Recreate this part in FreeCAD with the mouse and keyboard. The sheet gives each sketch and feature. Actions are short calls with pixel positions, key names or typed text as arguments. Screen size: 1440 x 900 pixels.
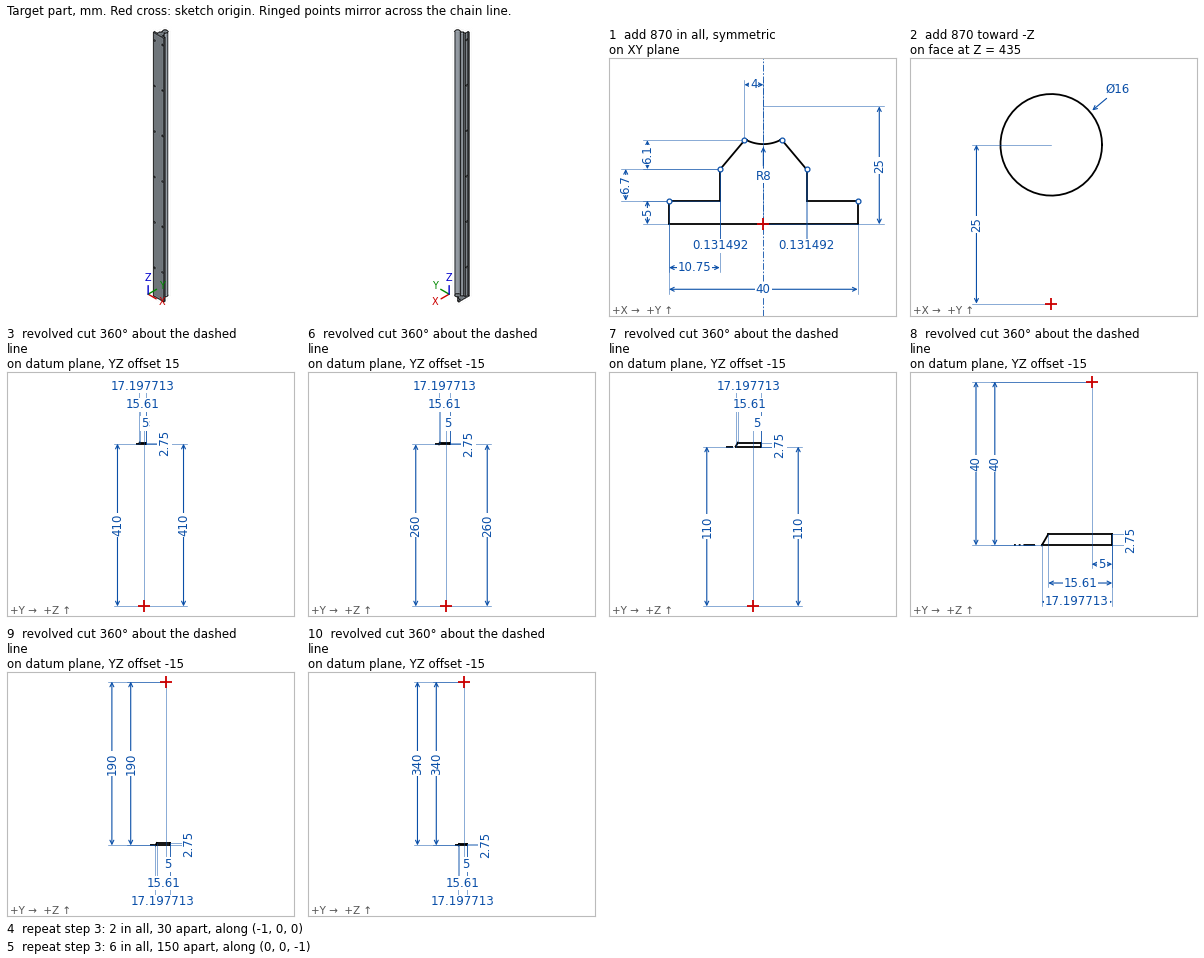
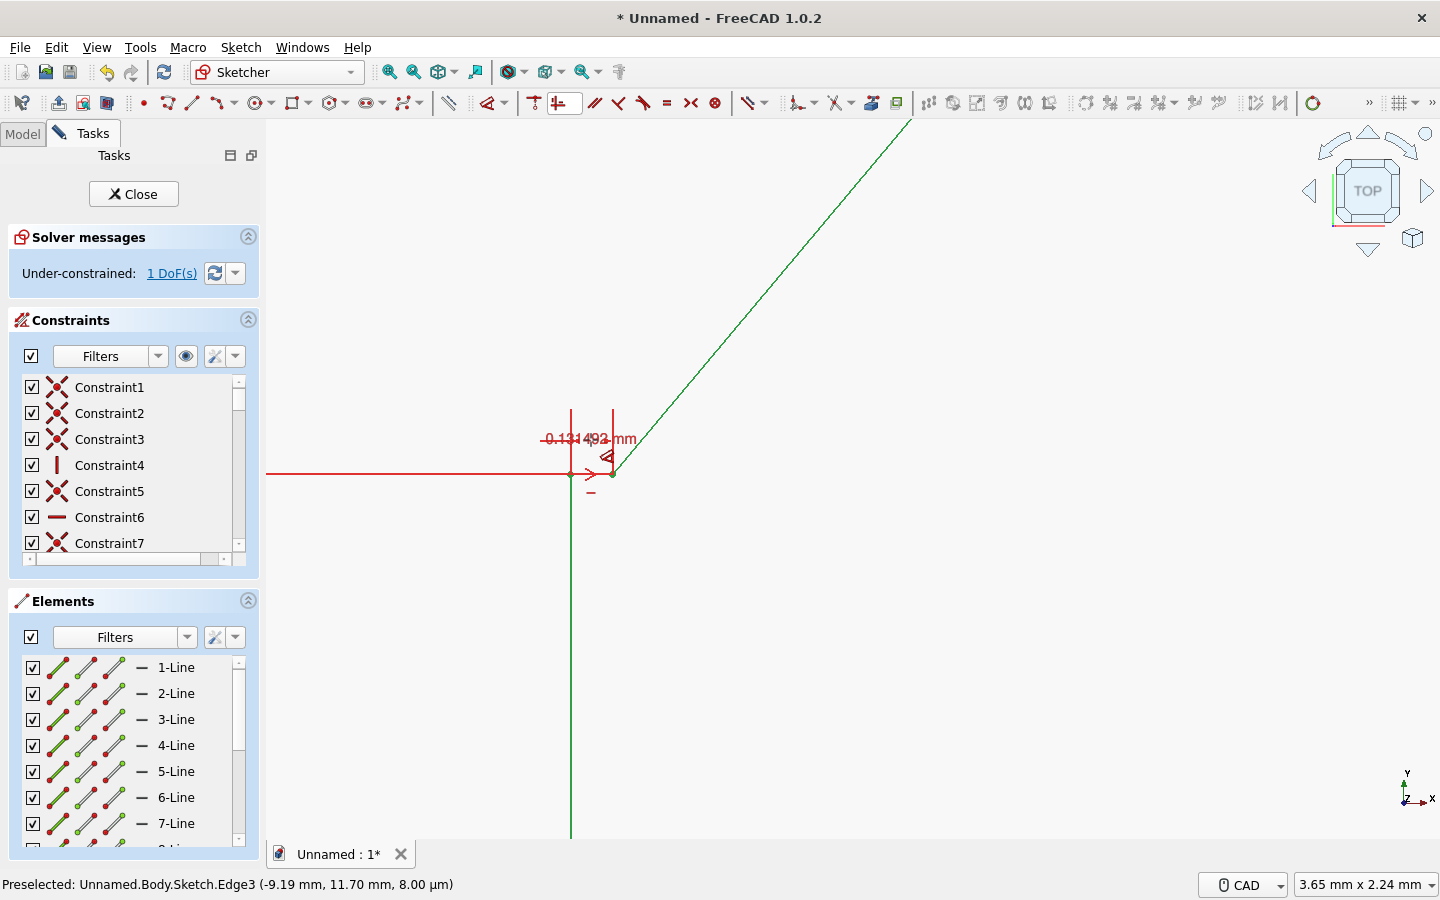
scroll(640, 432, down, 15)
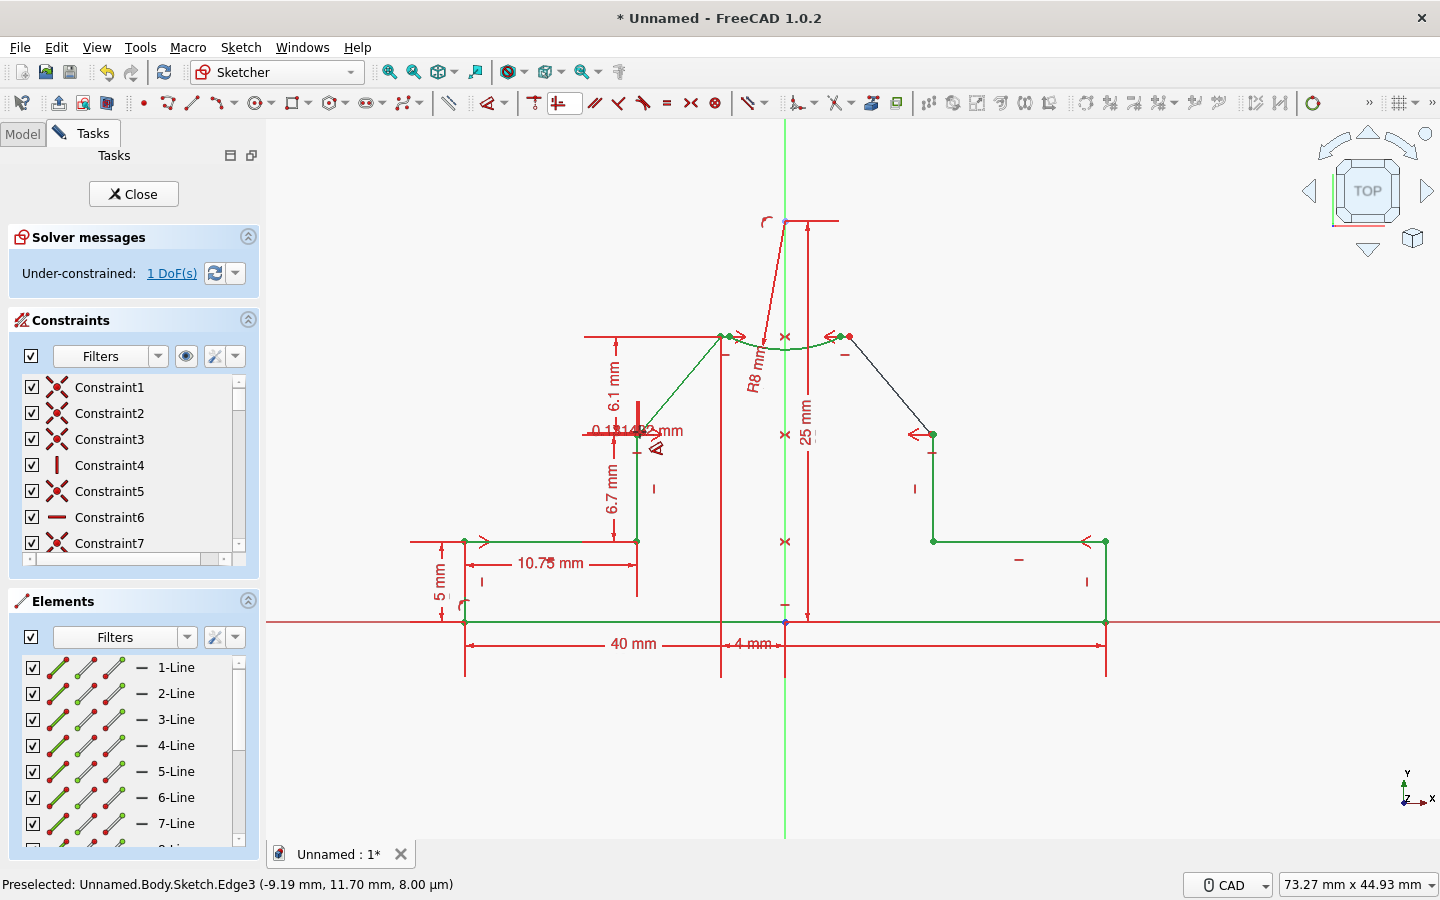
scroll(933, 435, up, 15)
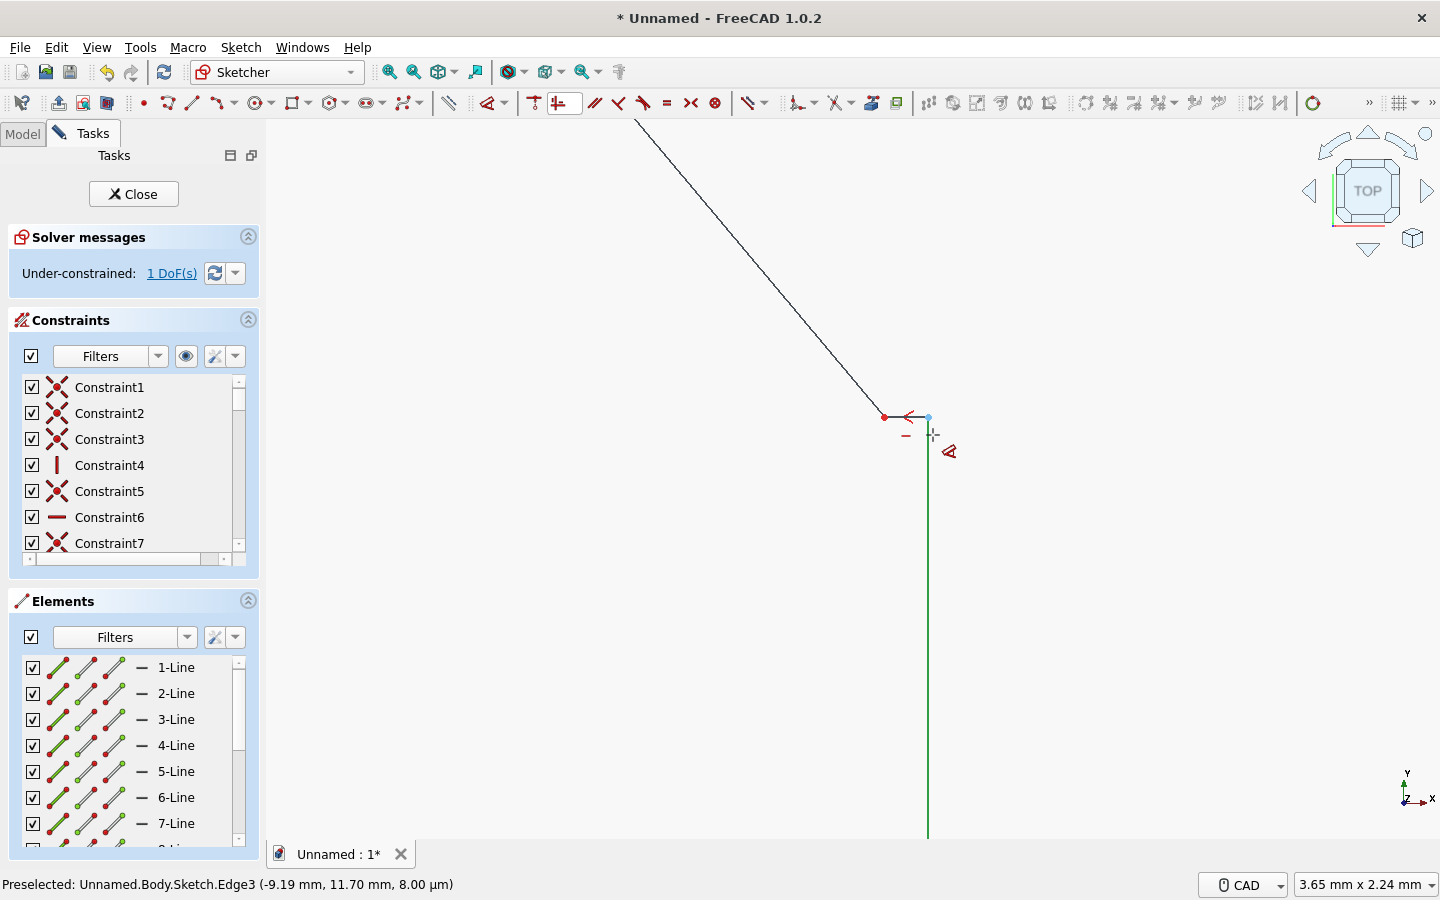
click(915, 417)
click(906, 383)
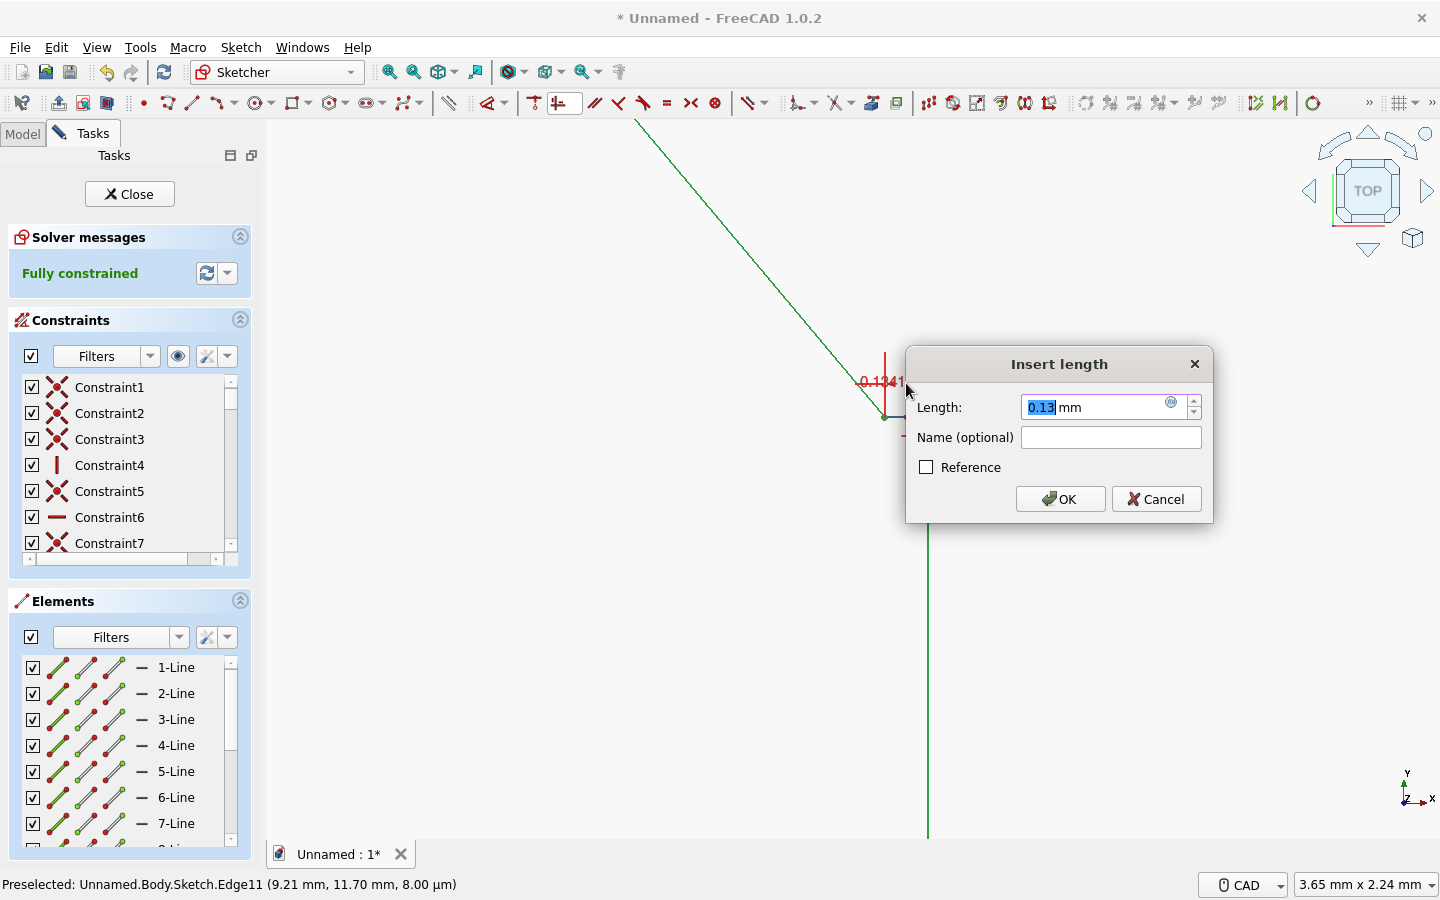
text(0.131492)
key(Return)
key(Escape)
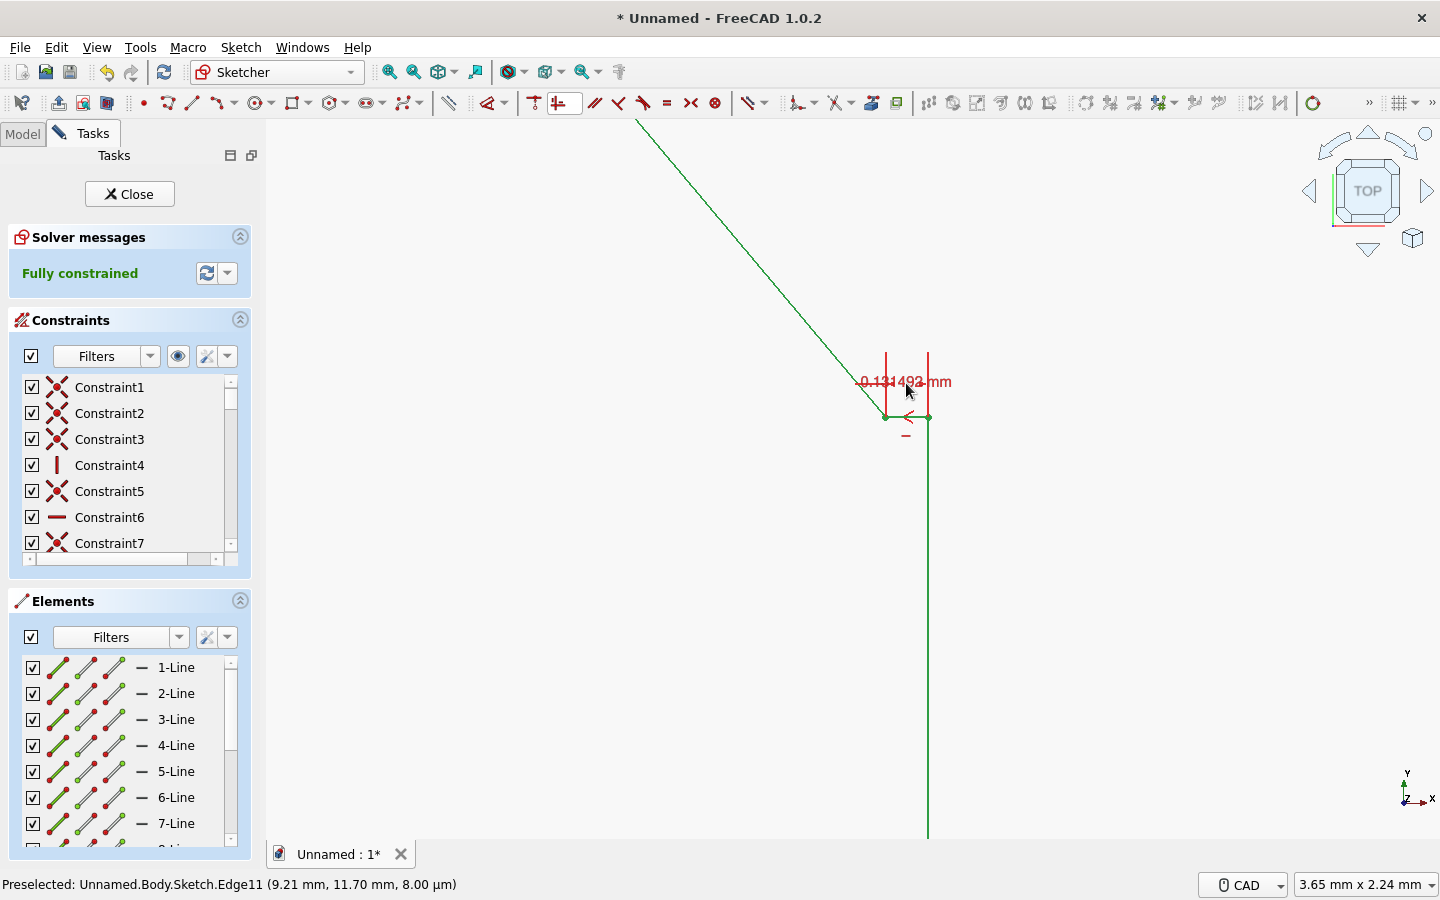
click(130, 194)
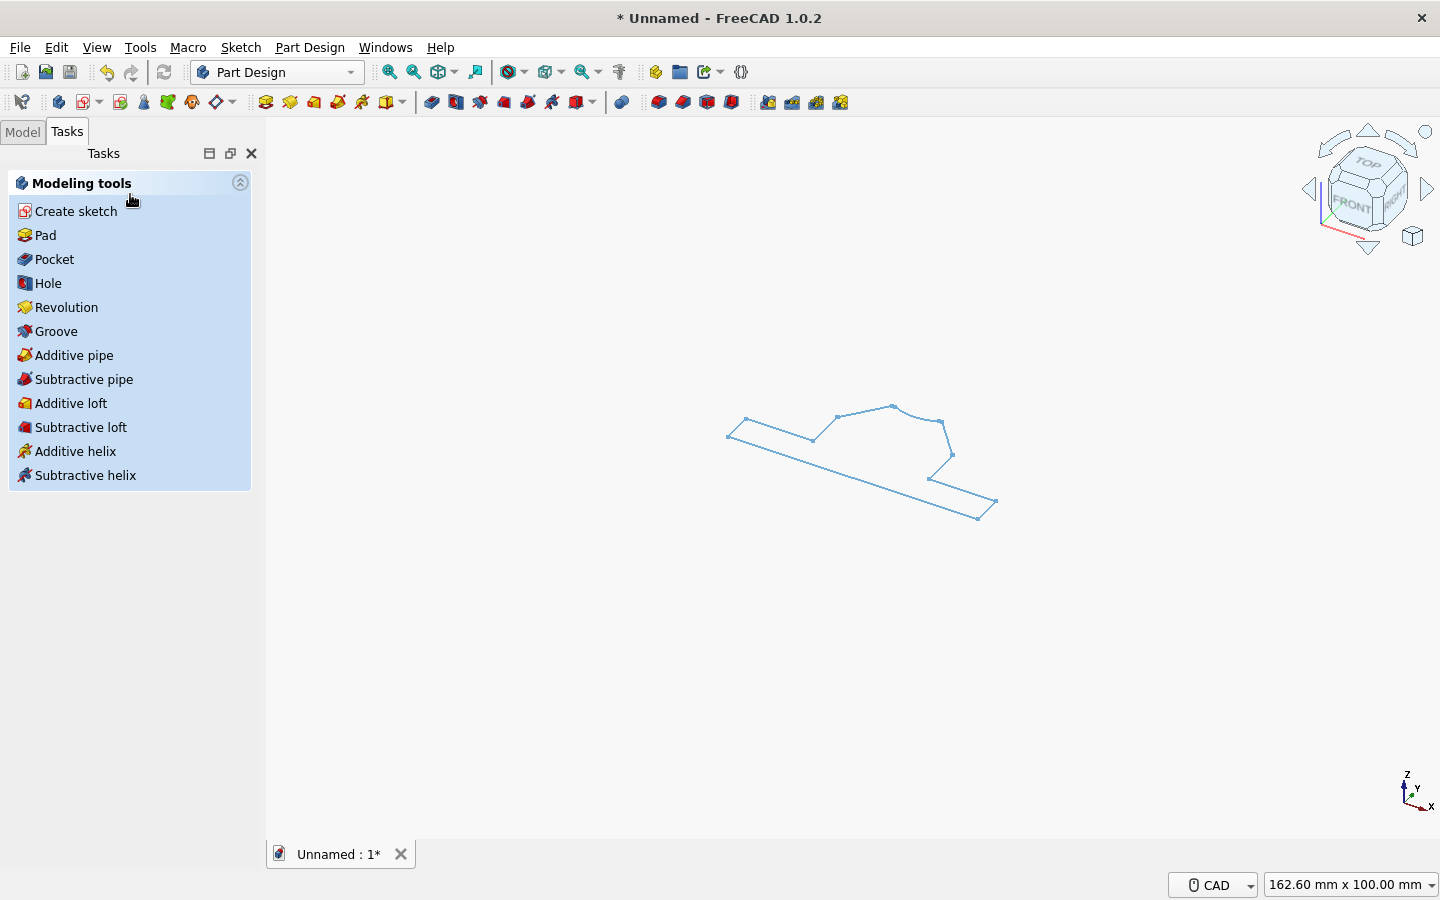
click(266, 102)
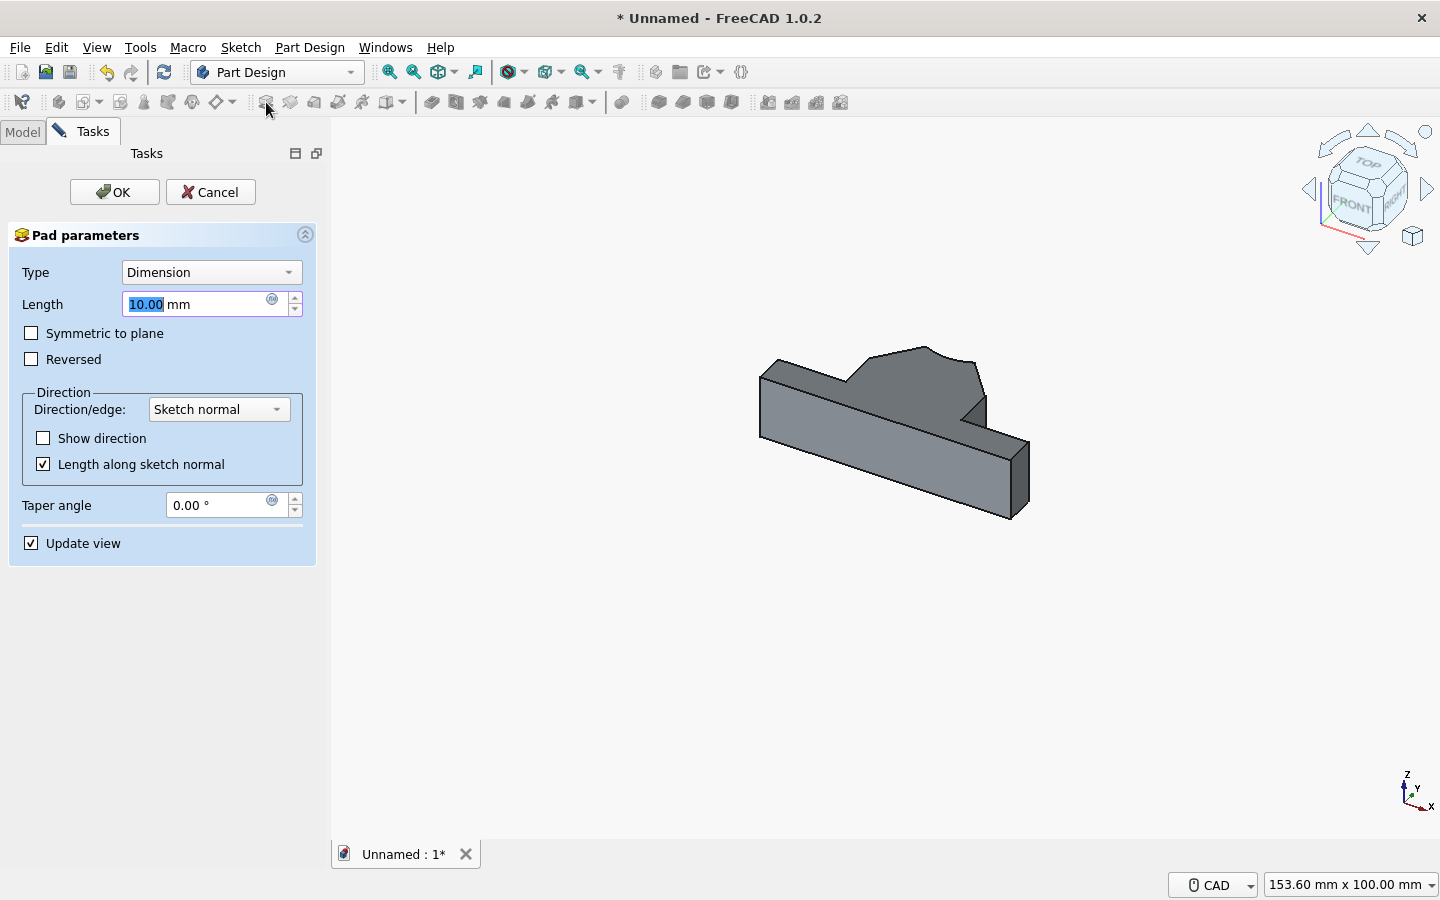
text(870)
key(Tab)